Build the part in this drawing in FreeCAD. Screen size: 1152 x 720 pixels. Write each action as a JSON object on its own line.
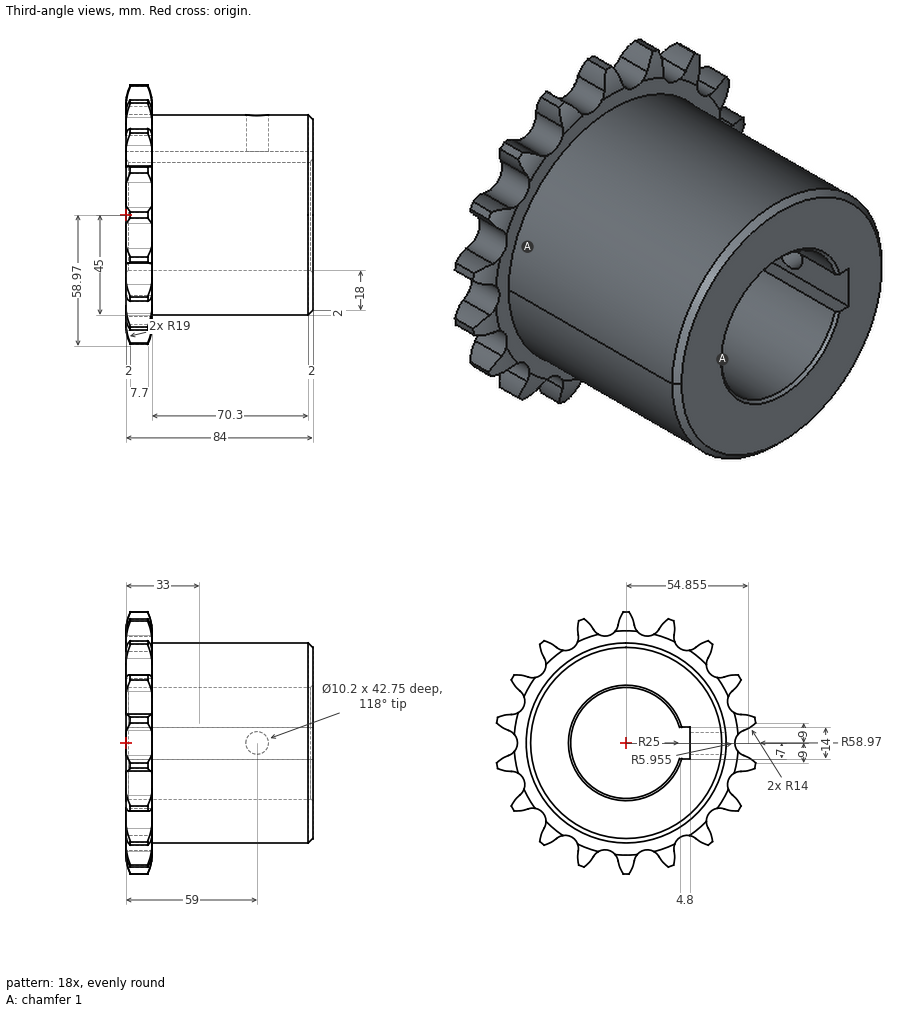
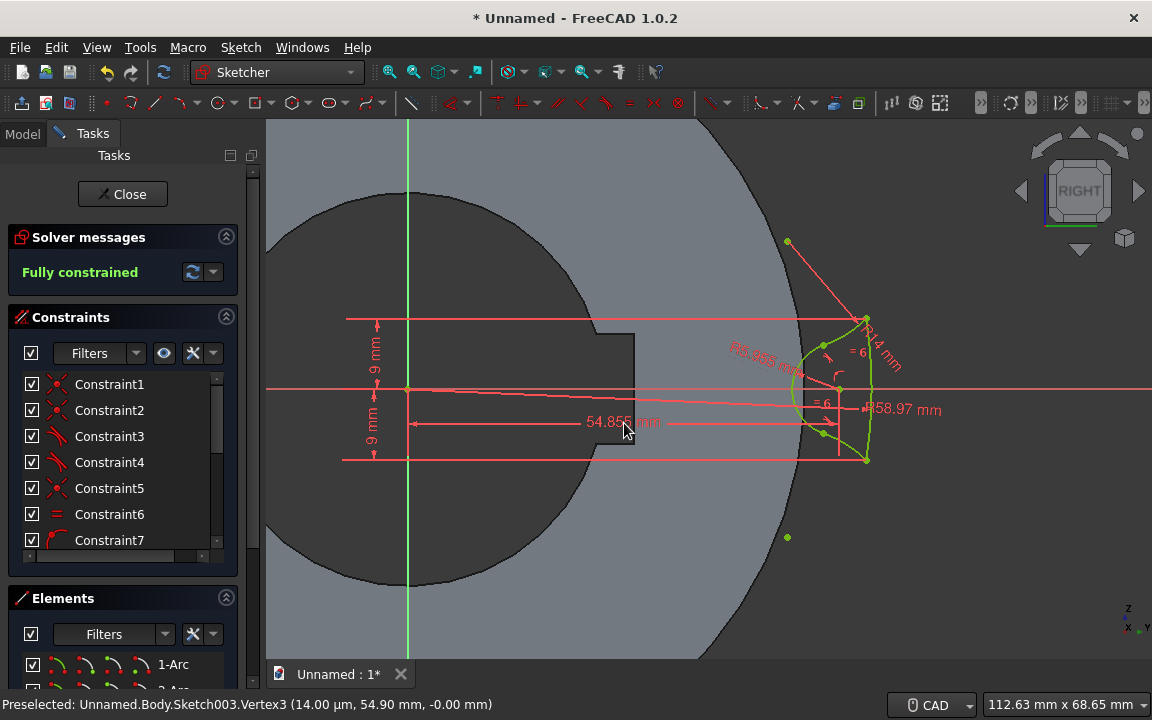
{"action": "left_click", "coordinate": [123, 194]}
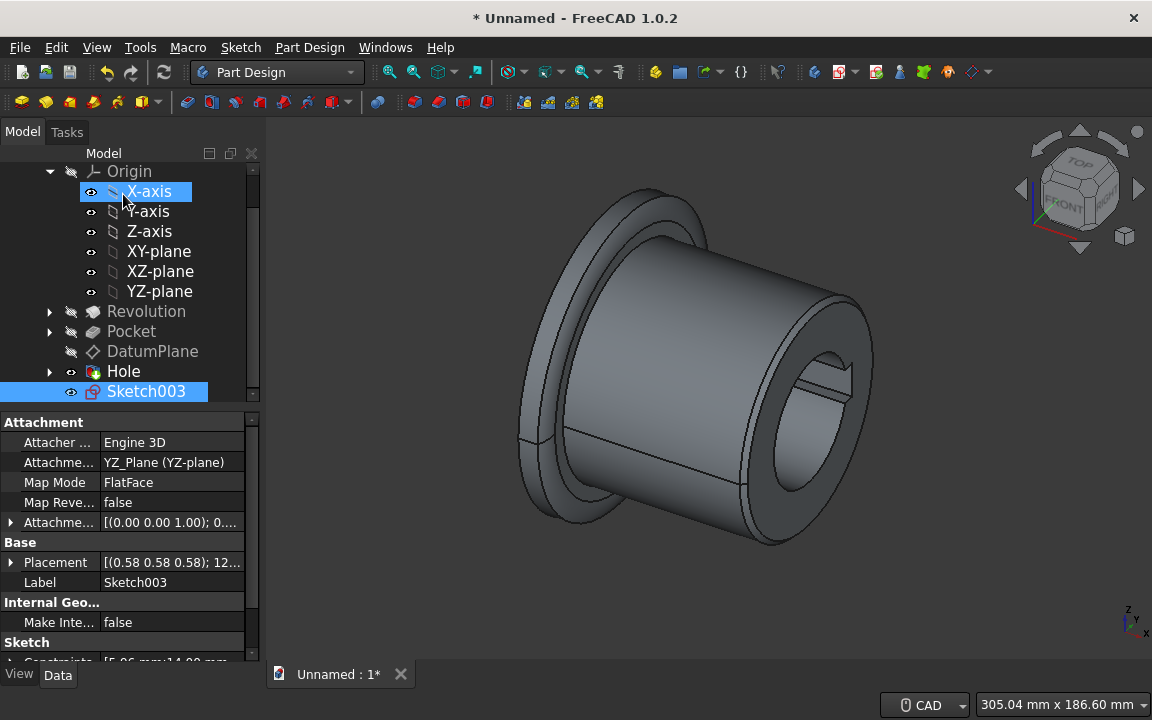
{"action": "left_click", "coordinate": [188, 102]}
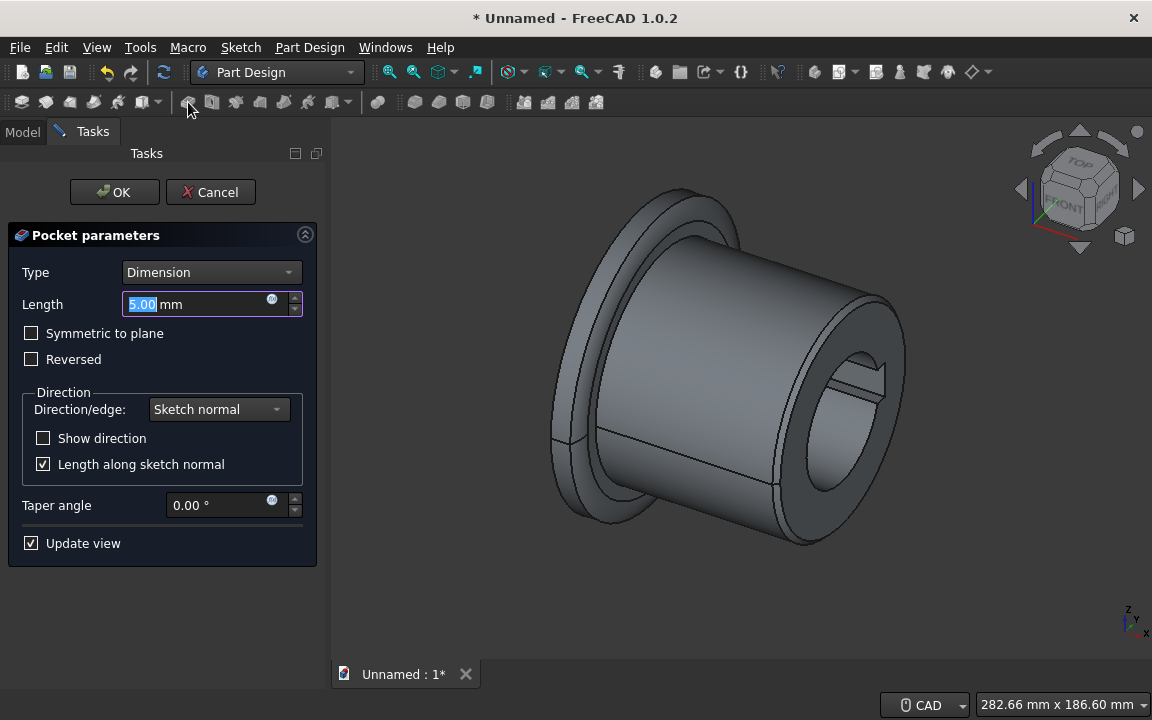
{"action": "type", "text": "33"}
{"action": "key", "text": "Tab"}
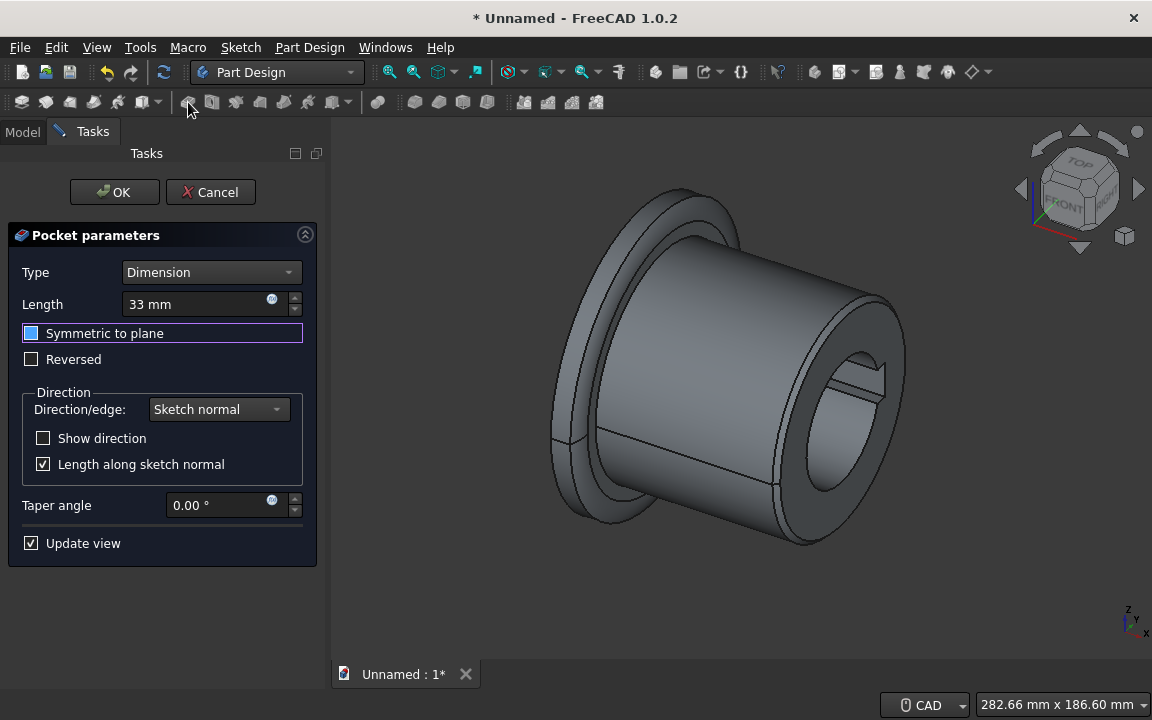
{"action": "left_click", "coordinate": [30, 359]}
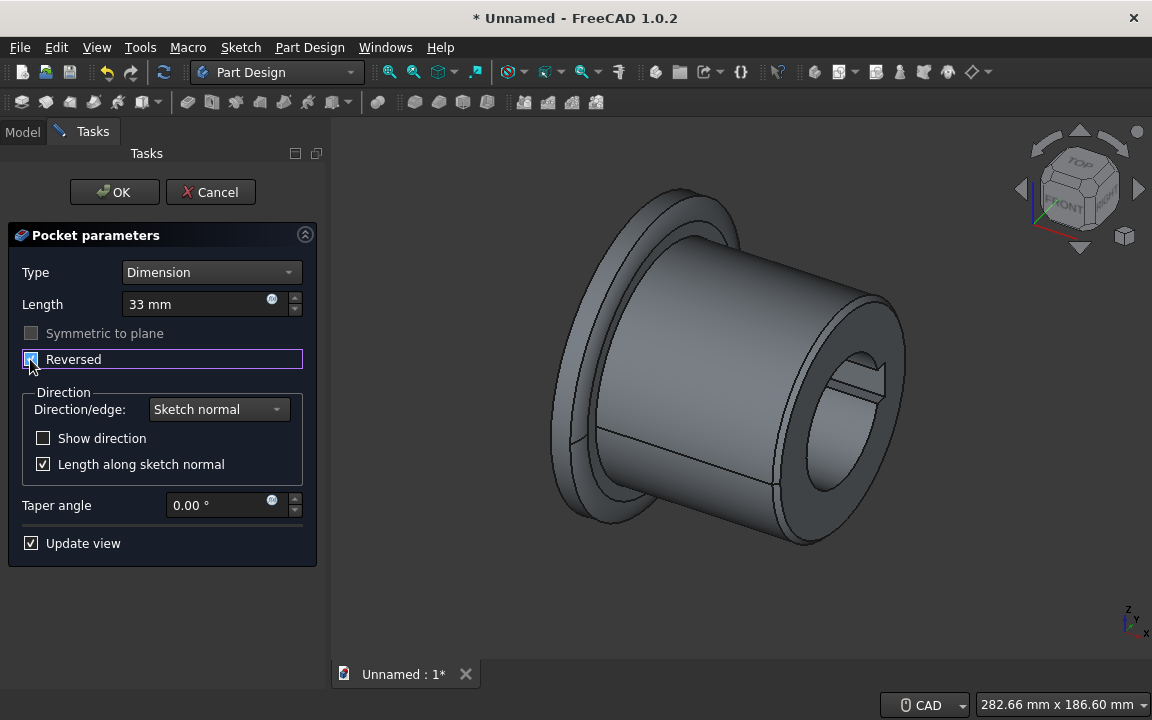
{"action": "left_click", "coordinate": [115, 192]}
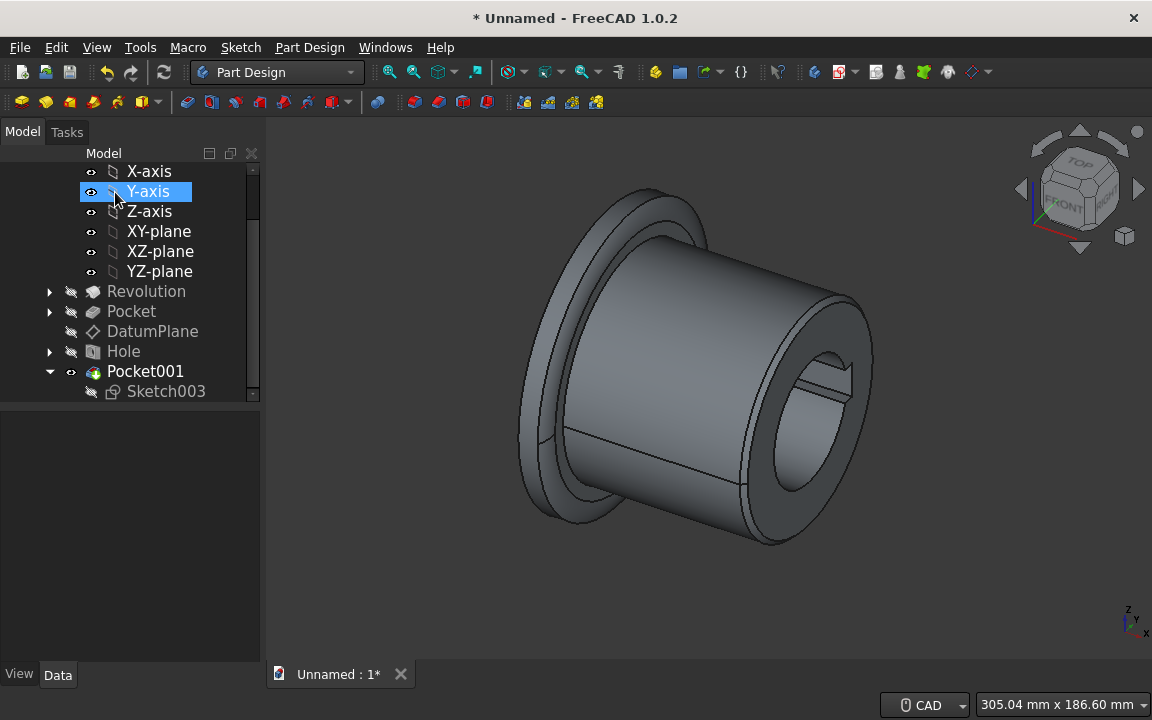
{"action": "left_click", "coordinate": [116, 372]}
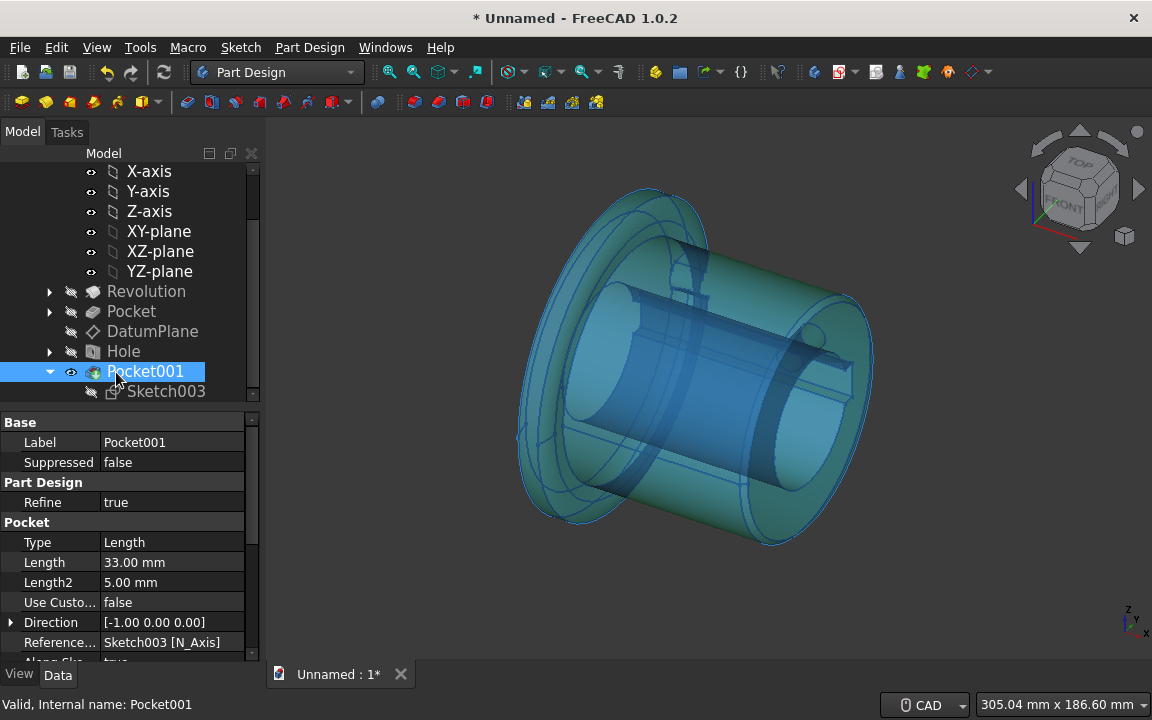
{"action": "left_click", "coordinate": [572, 102]}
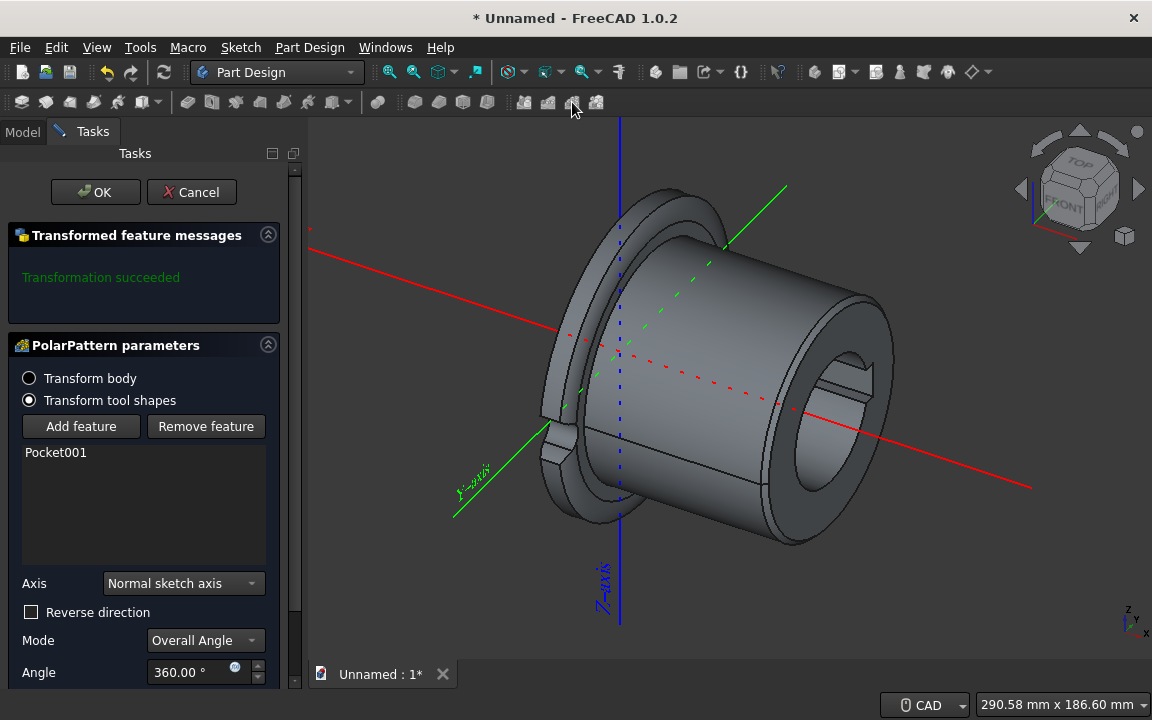
{"action": "left_click", "coordinate": [184, 584]}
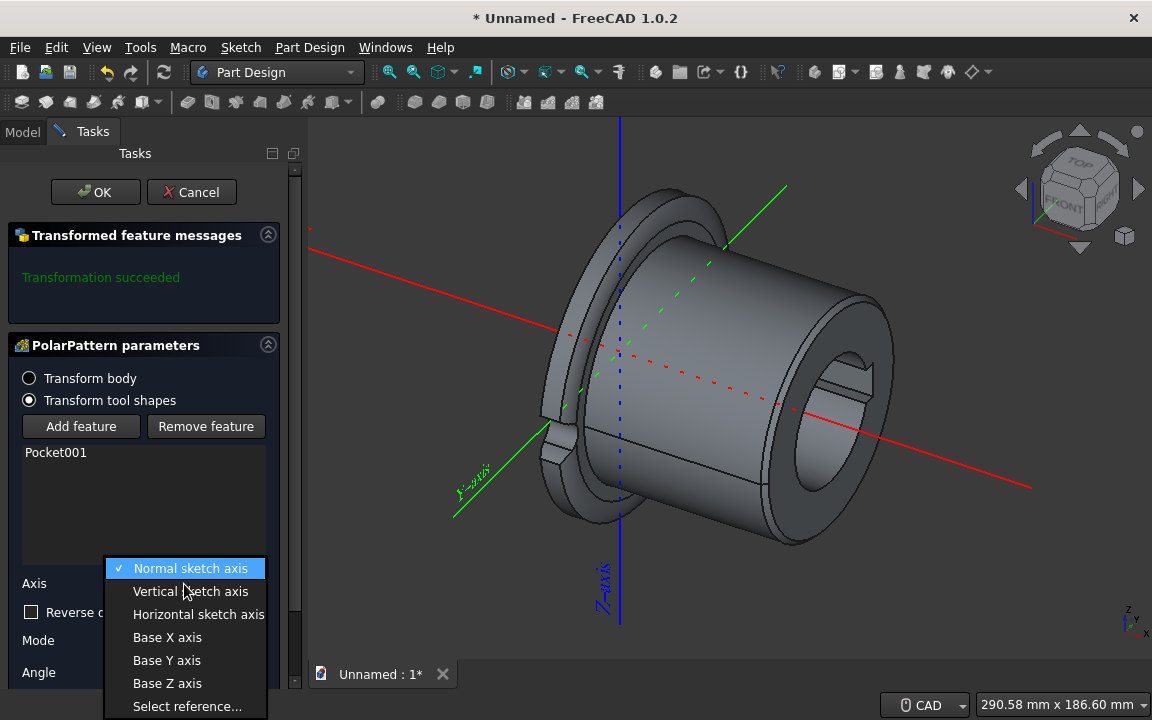
{"action": "left_click", "coordinate": [184, 638]}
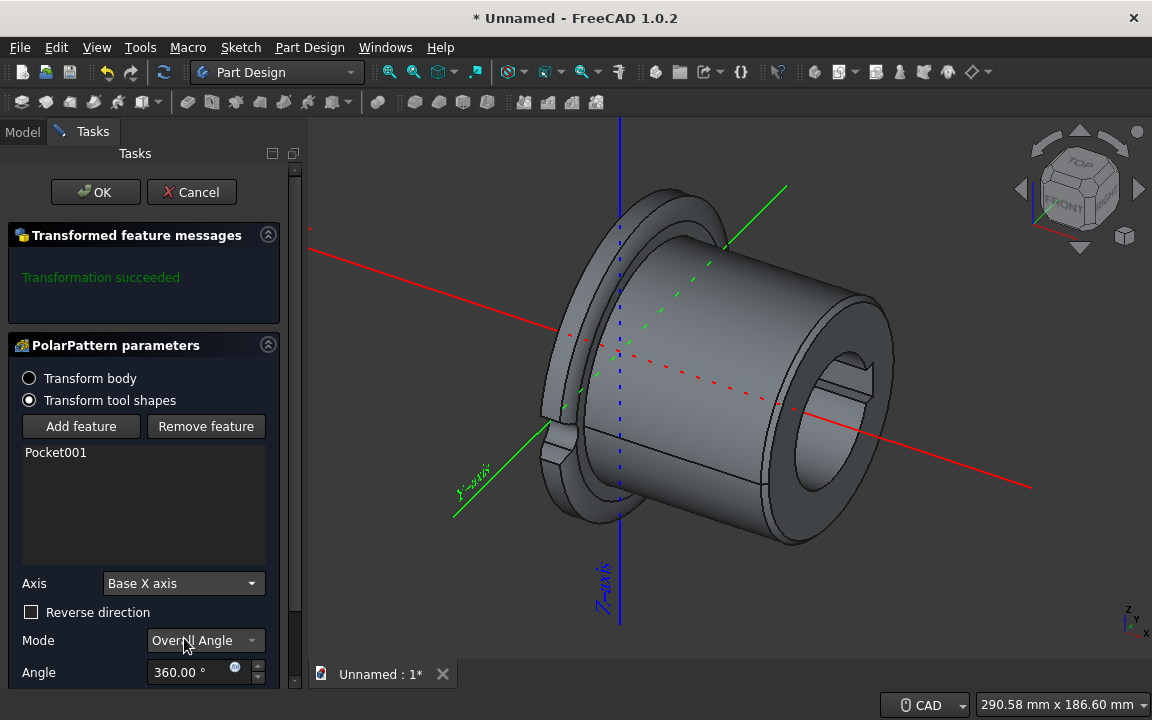
{"action": "scroll", "coordinate": [295, 426], "scroll_direction": "down", "scroll_amount": 2}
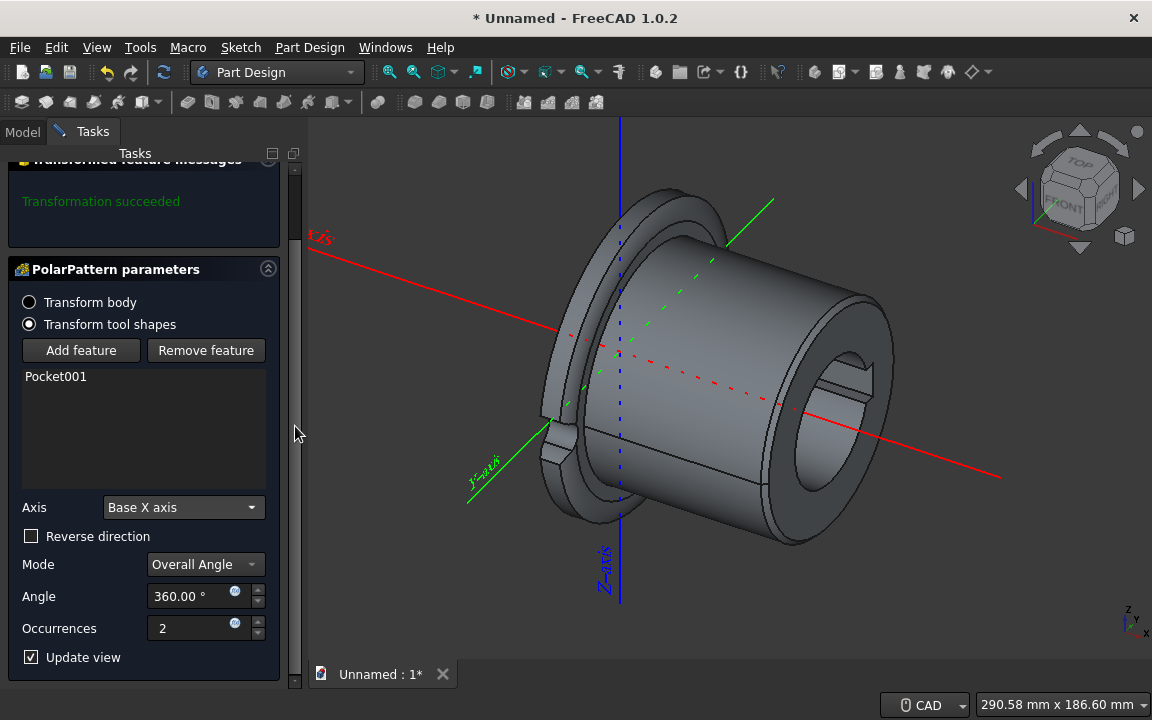
{"action": "triple_click", "coordinate": [198, 628]}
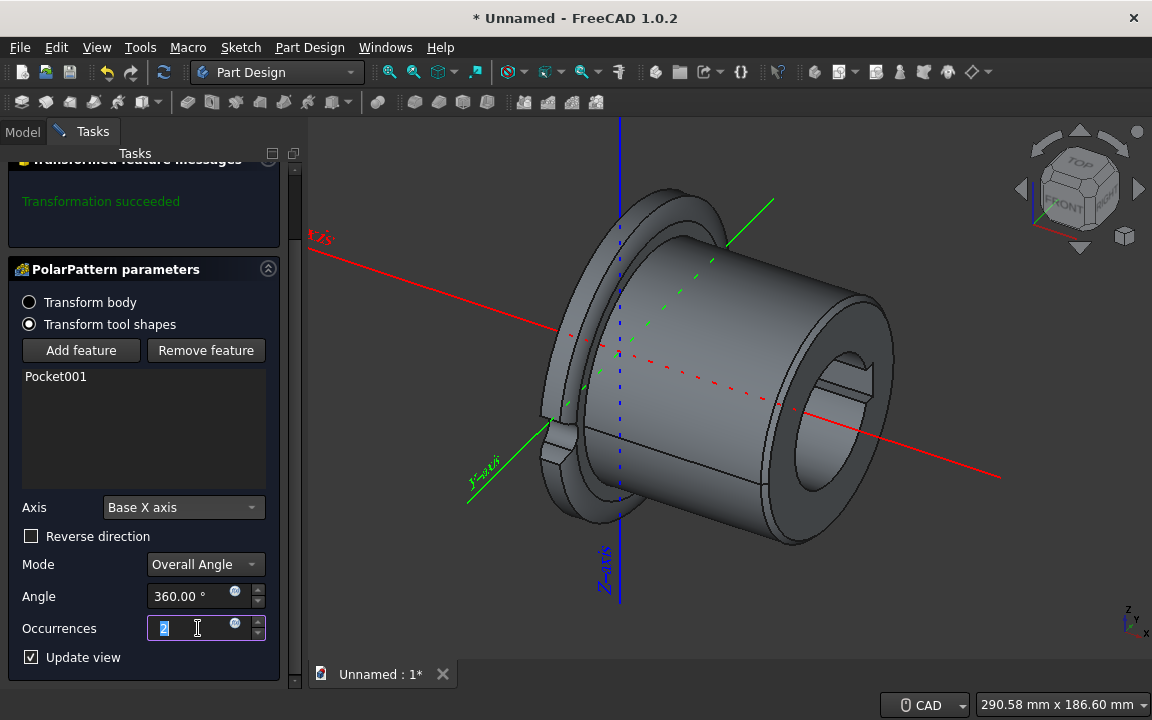
{"action": "type", "text": "18"}
{"action": "key", "text": "Tab"}